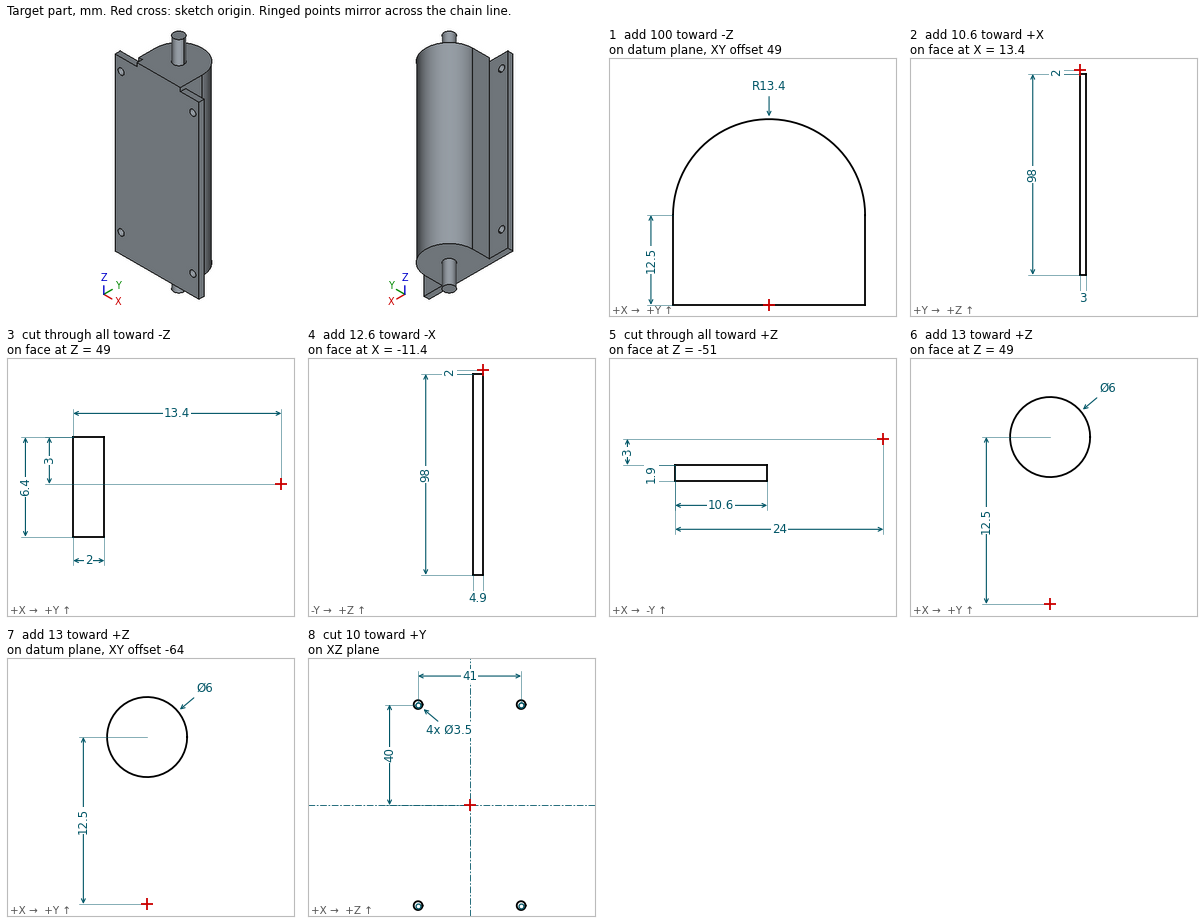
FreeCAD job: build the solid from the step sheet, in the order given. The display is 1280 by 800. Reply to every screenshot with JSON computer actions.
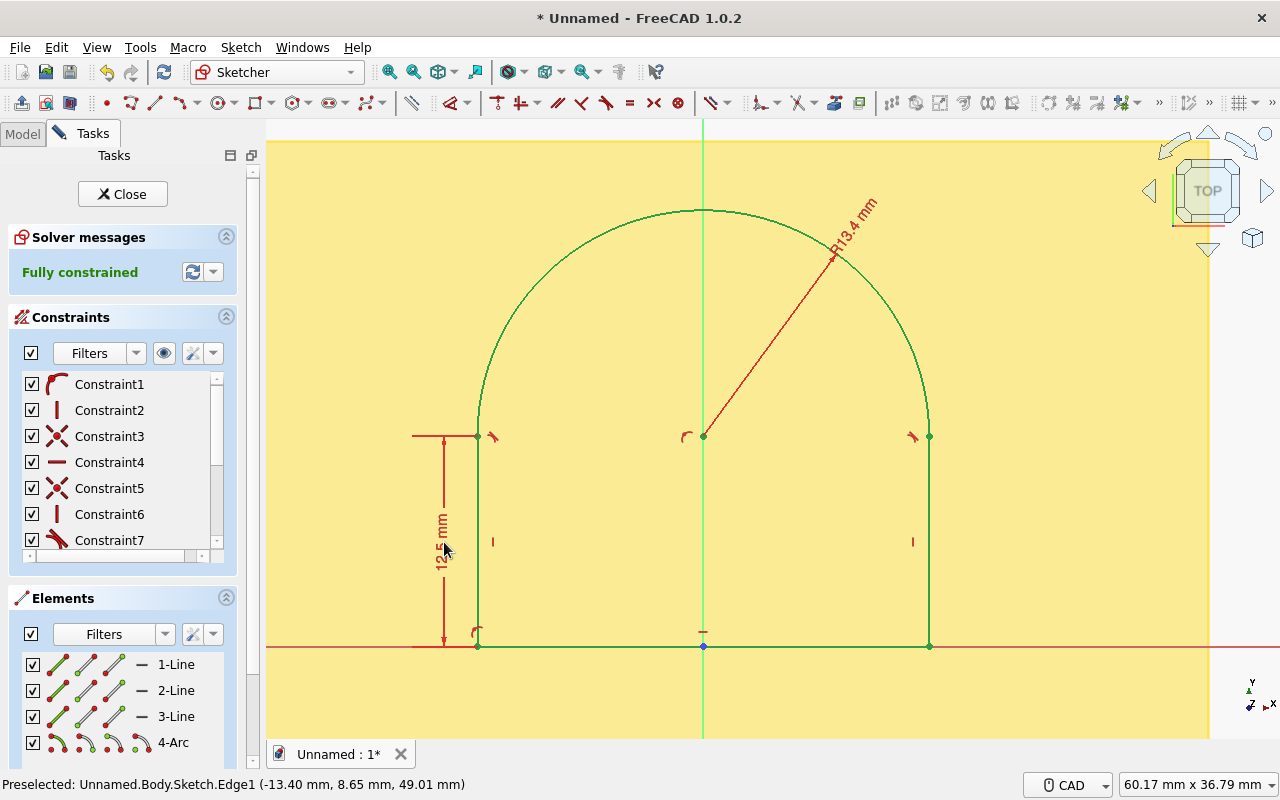
{"action": "left_click", "coordinate": [123, 194]}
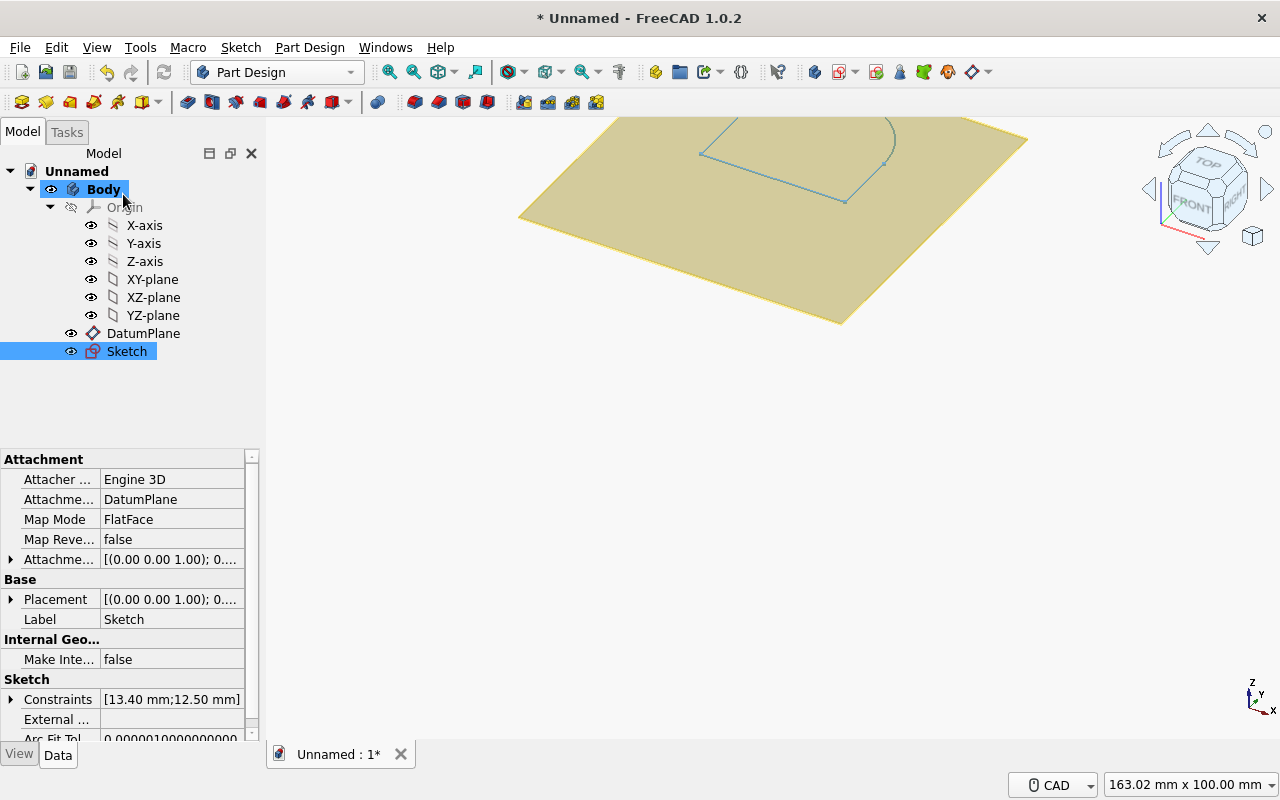
{"action": "left_click", "coordinate": [22, 102]}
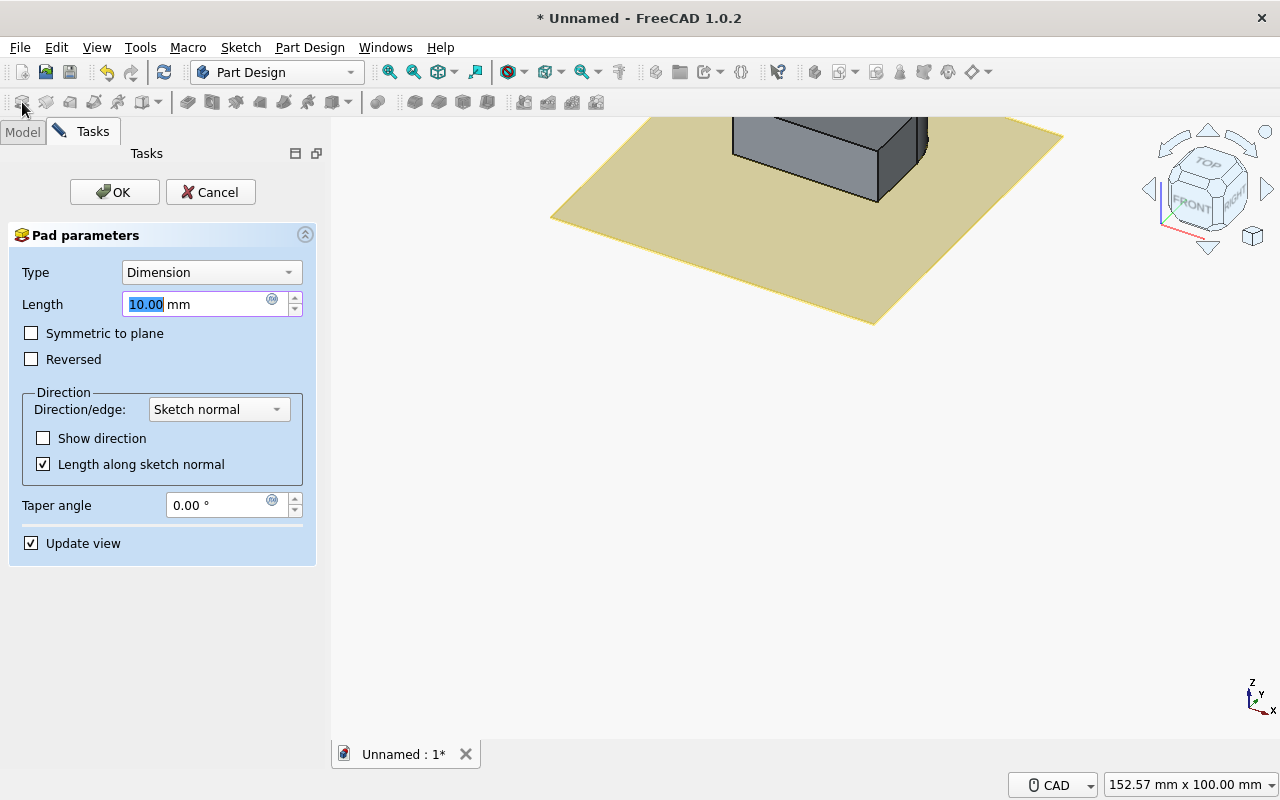
{"action": "type", "text": "100"}
{"action": "key", "text": "Tab"}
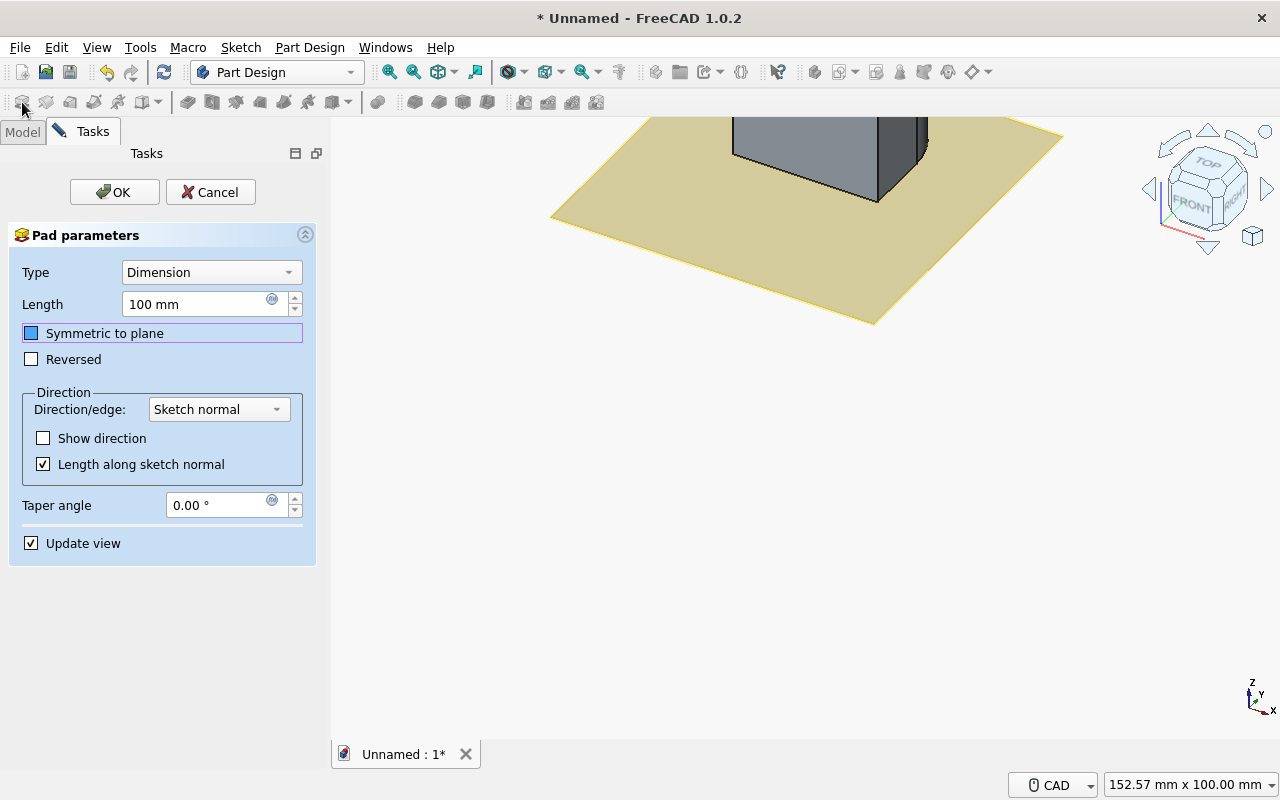
{"action": "left_click", "coordinate": [30, 359]}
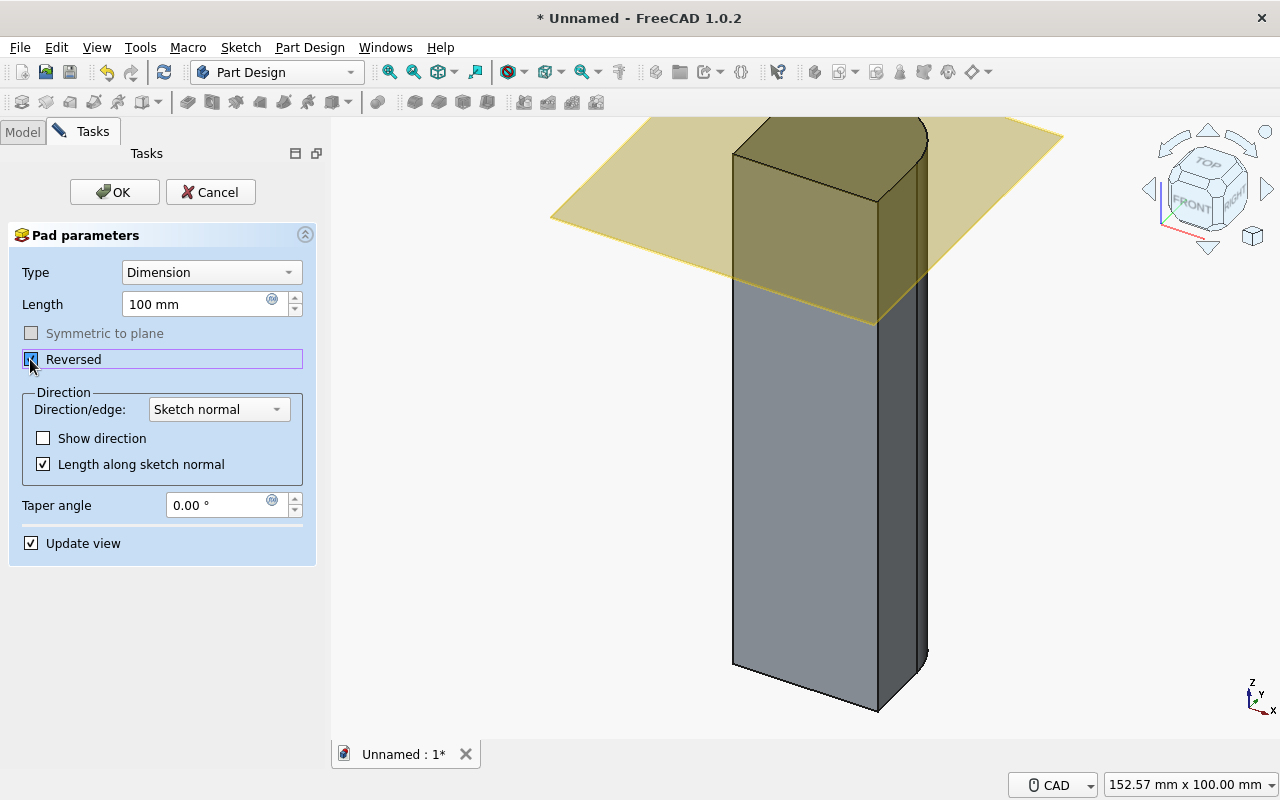
{"action": "left_click", "coordinate": [115, 192]}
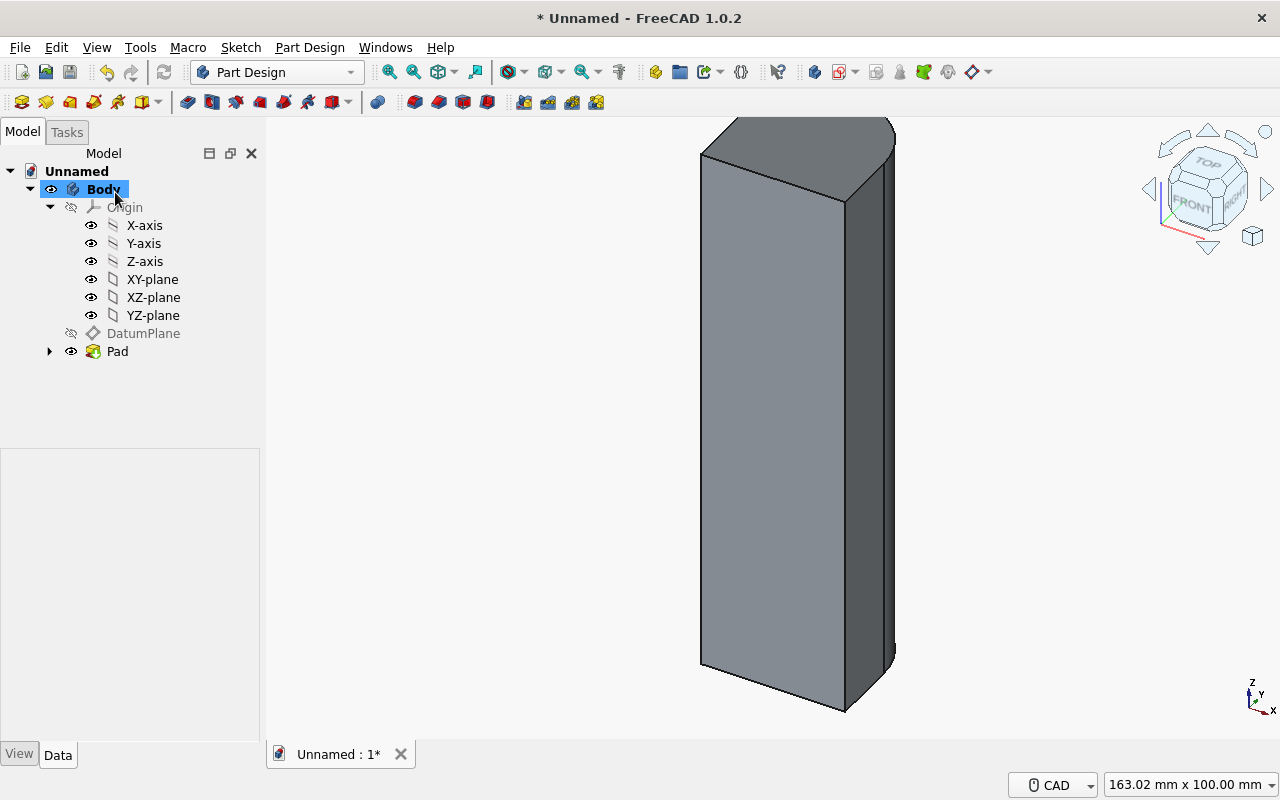
{"action": "left_click", "coordinate": [390, 72]}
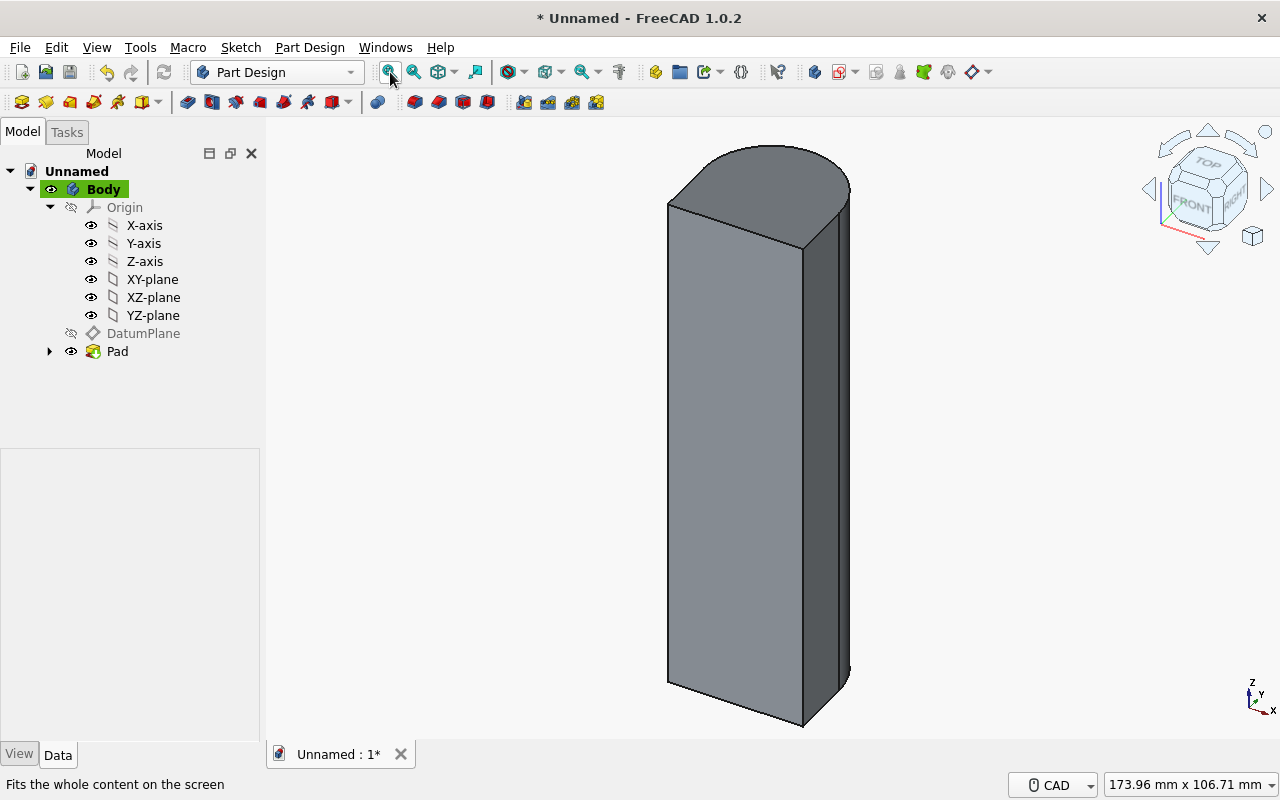
{"action": "left_click", "coordinate": [821, 264]}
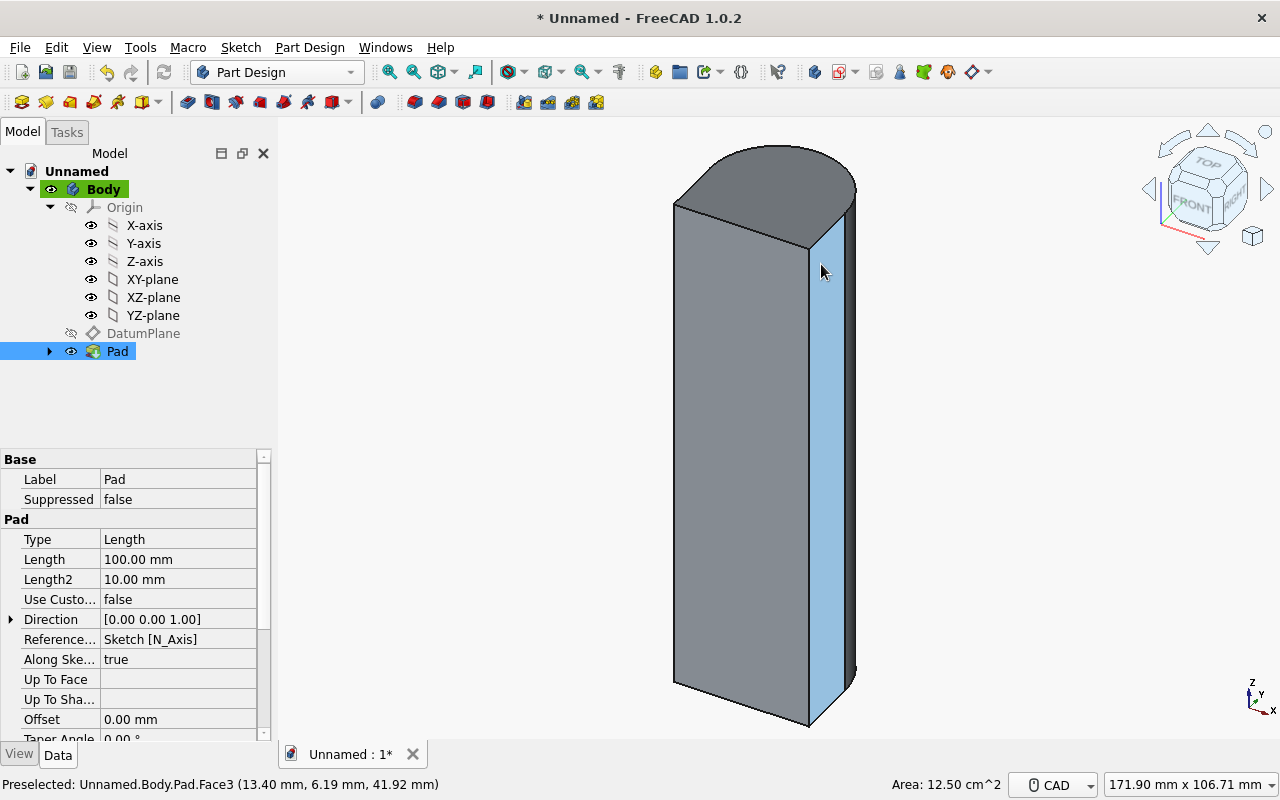
{"action": "left_click", "coordinate": [840, 72]}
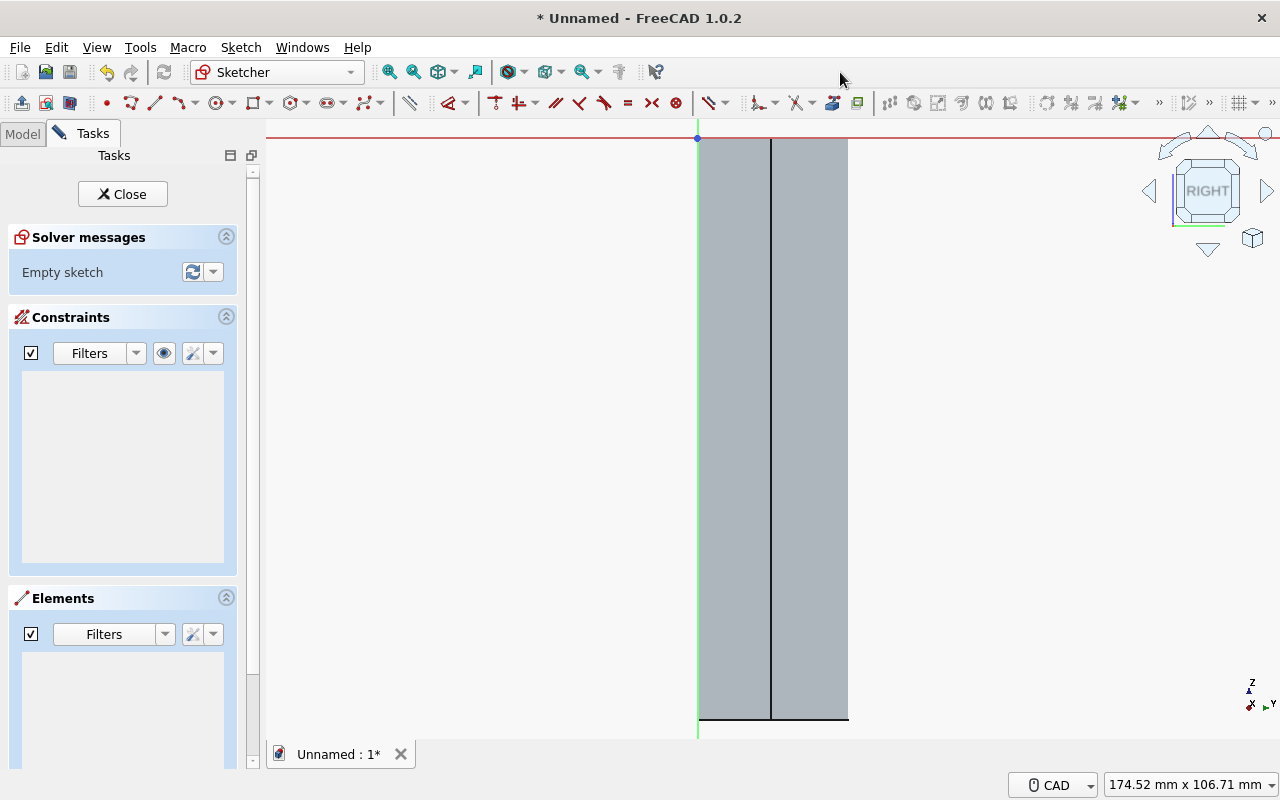
{"action": "scroll", "coordinate": [700, 429], "scroll_direction": "down", "scroll_amount": 2}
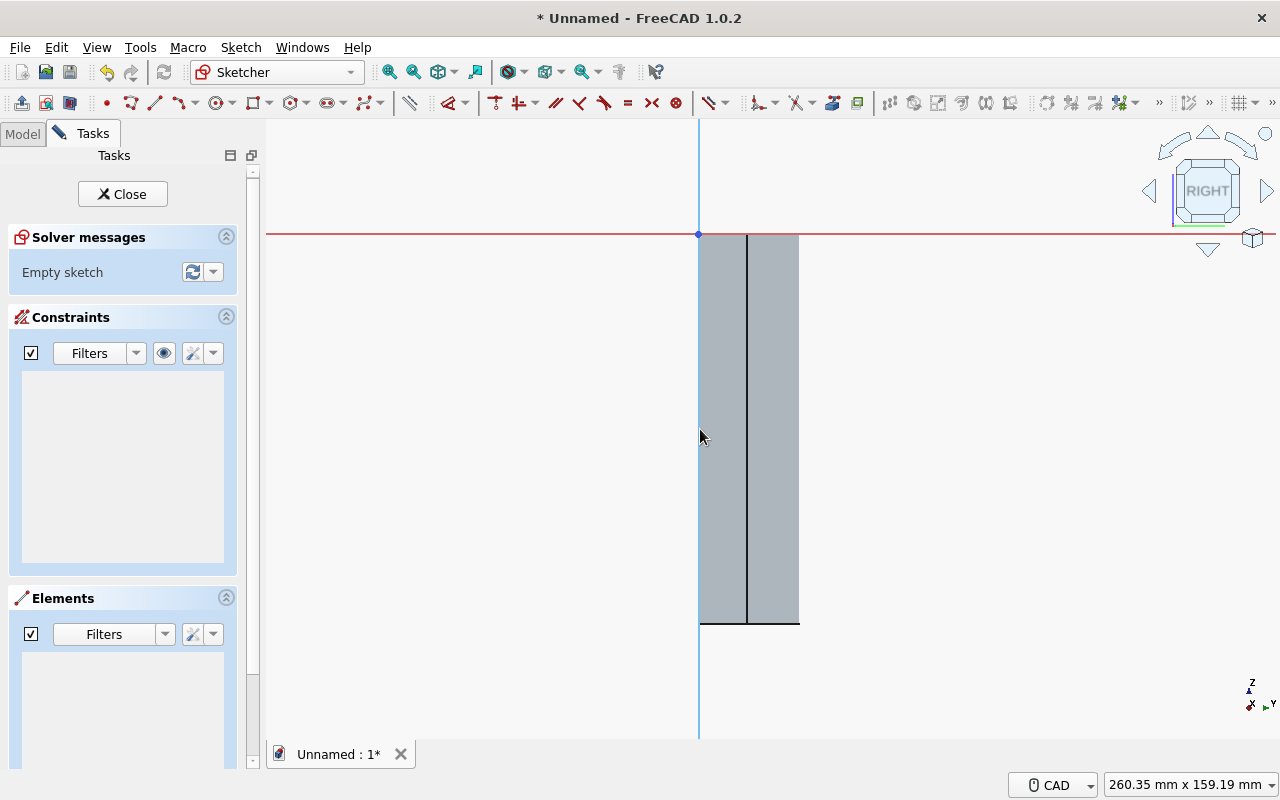
{"action": "left_click", "coordinate": [254, 104]}